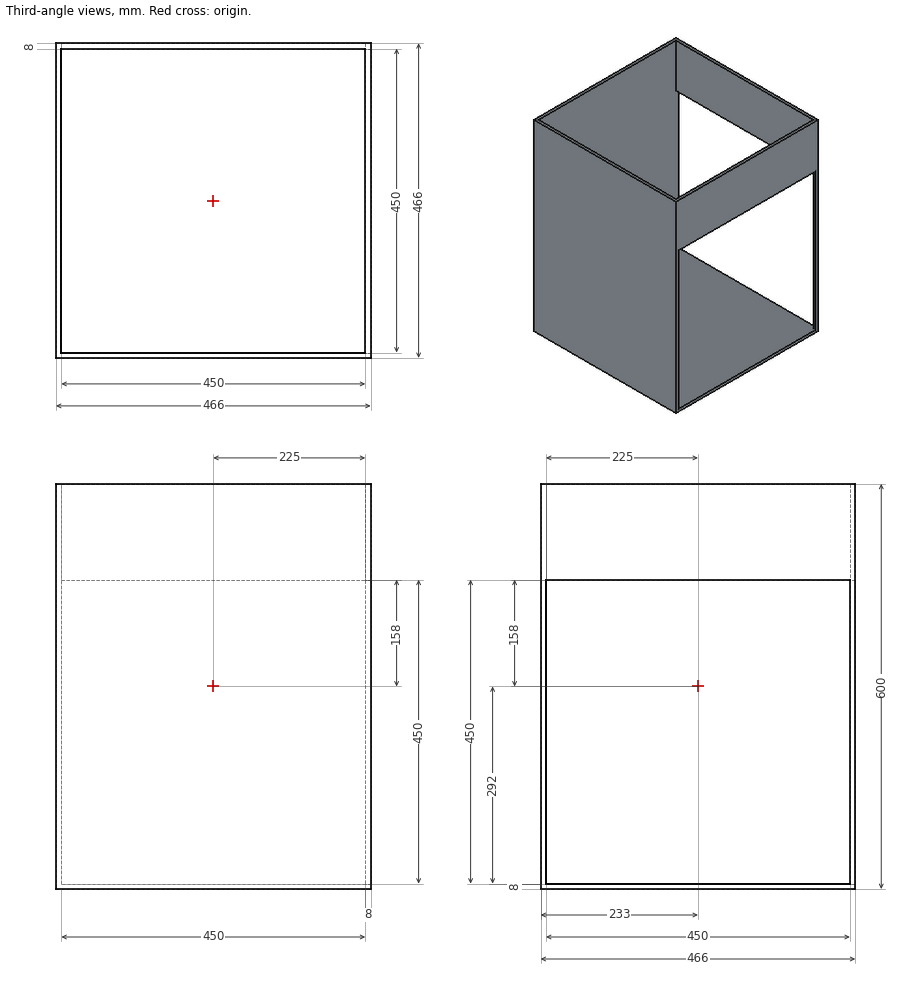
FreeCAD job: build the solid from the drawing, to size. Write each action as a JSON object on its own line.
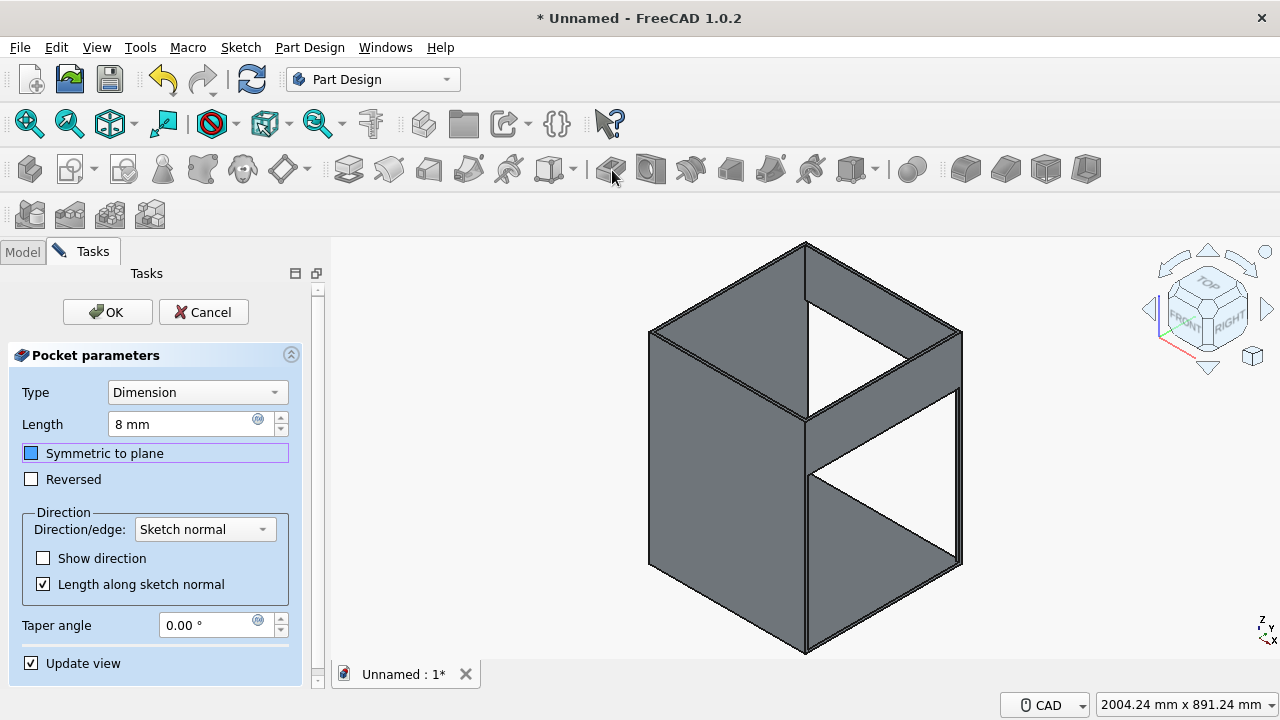
{"action": "left_click", "coordinate": [108, 312]}